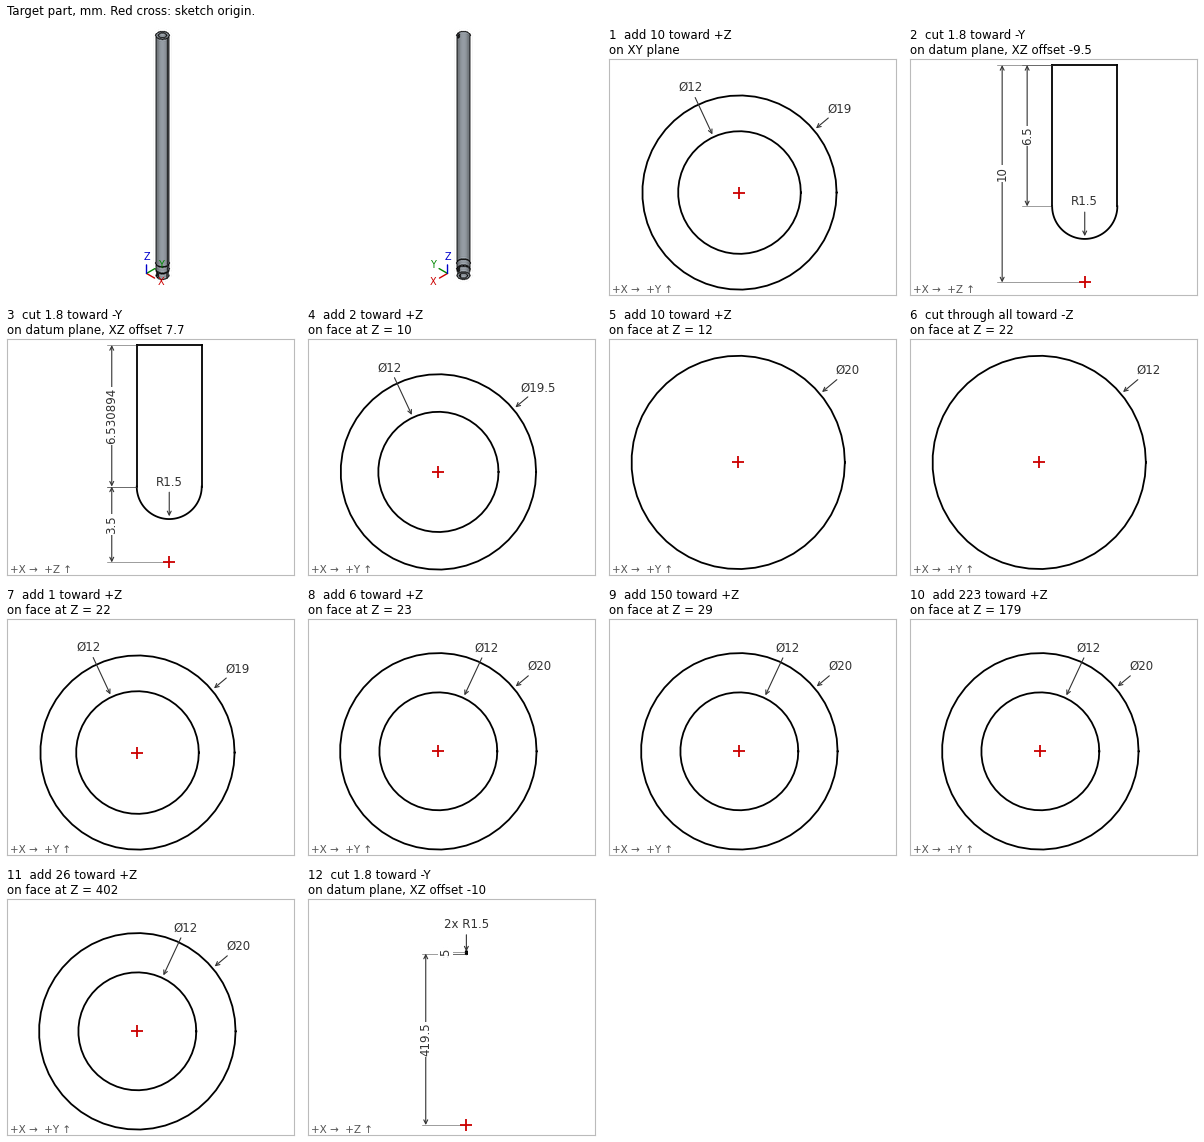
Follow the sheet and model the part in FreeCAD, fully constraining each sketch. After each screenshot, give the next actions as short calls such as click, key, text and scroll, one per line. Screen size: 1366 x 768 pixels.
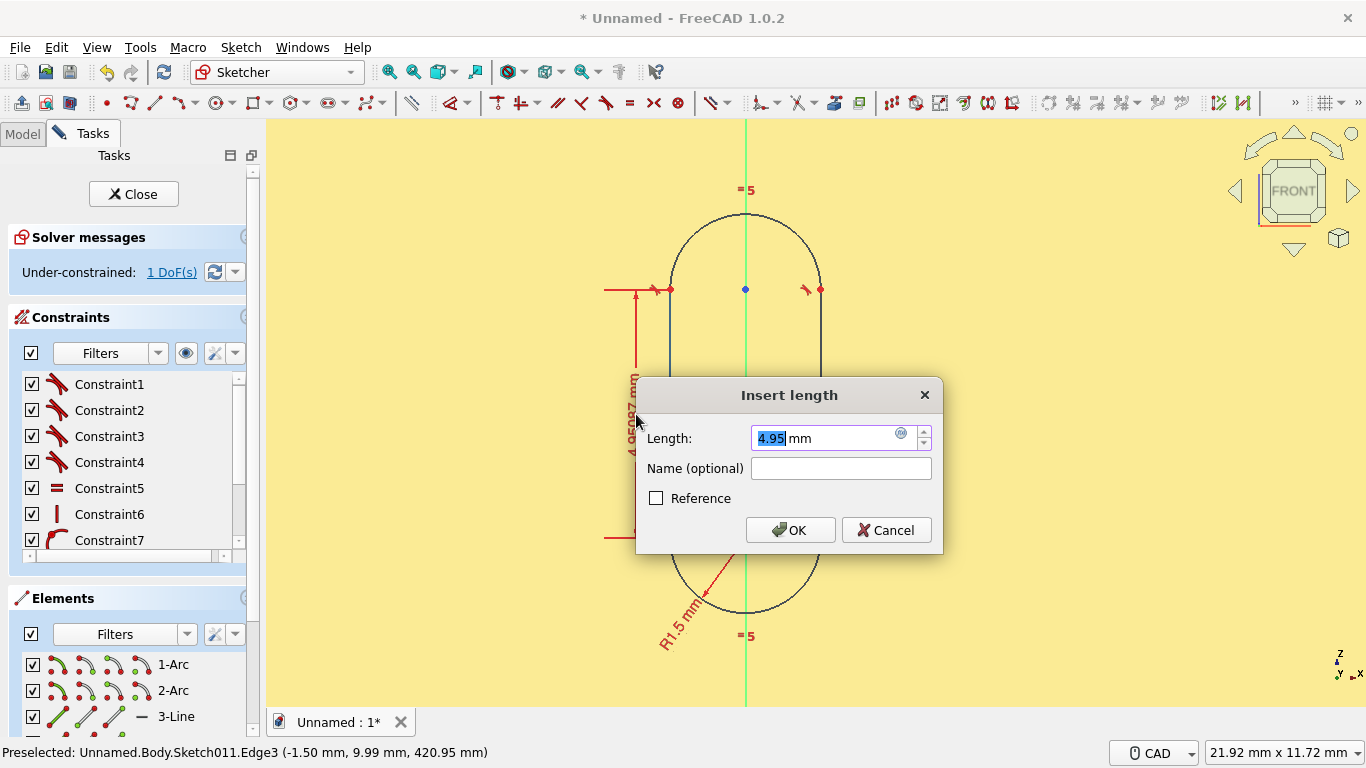
text(5)
key(Return)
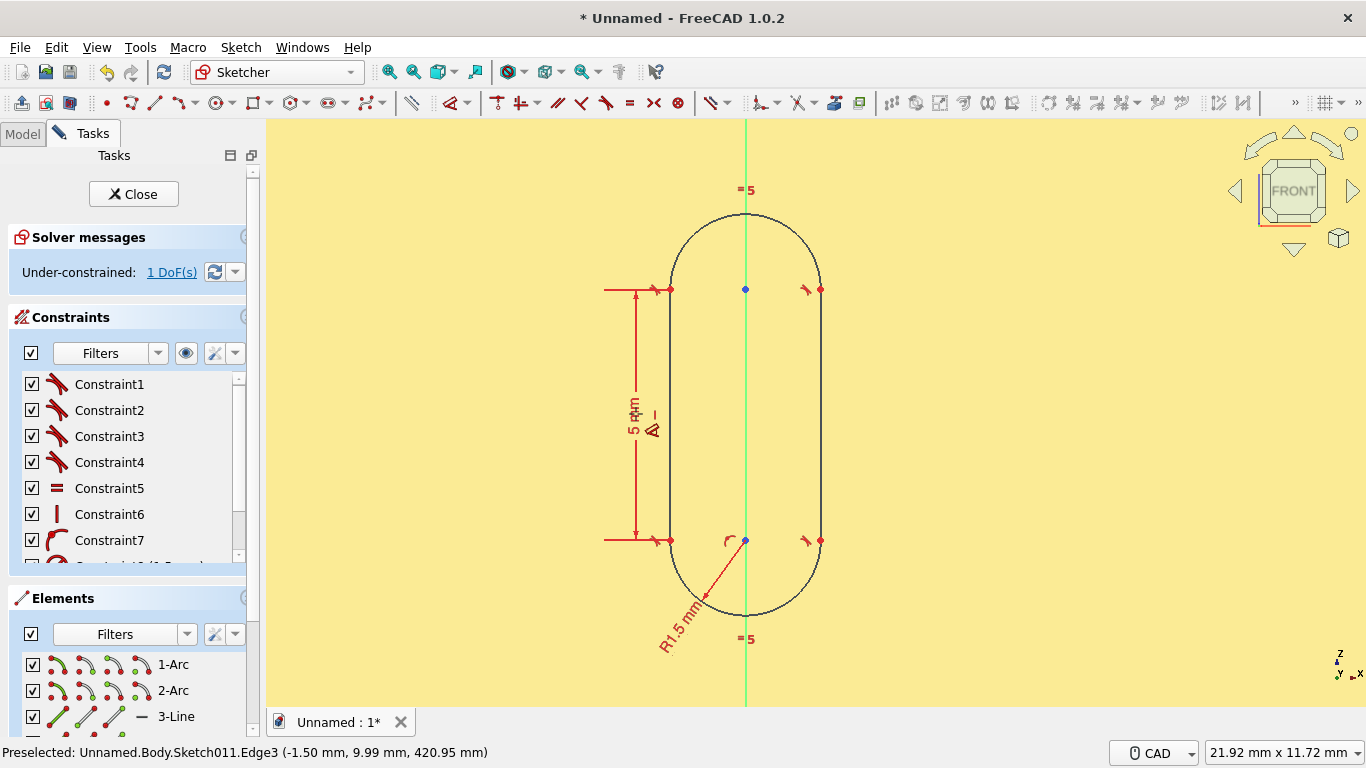
click(670, 540)
click(636, 578)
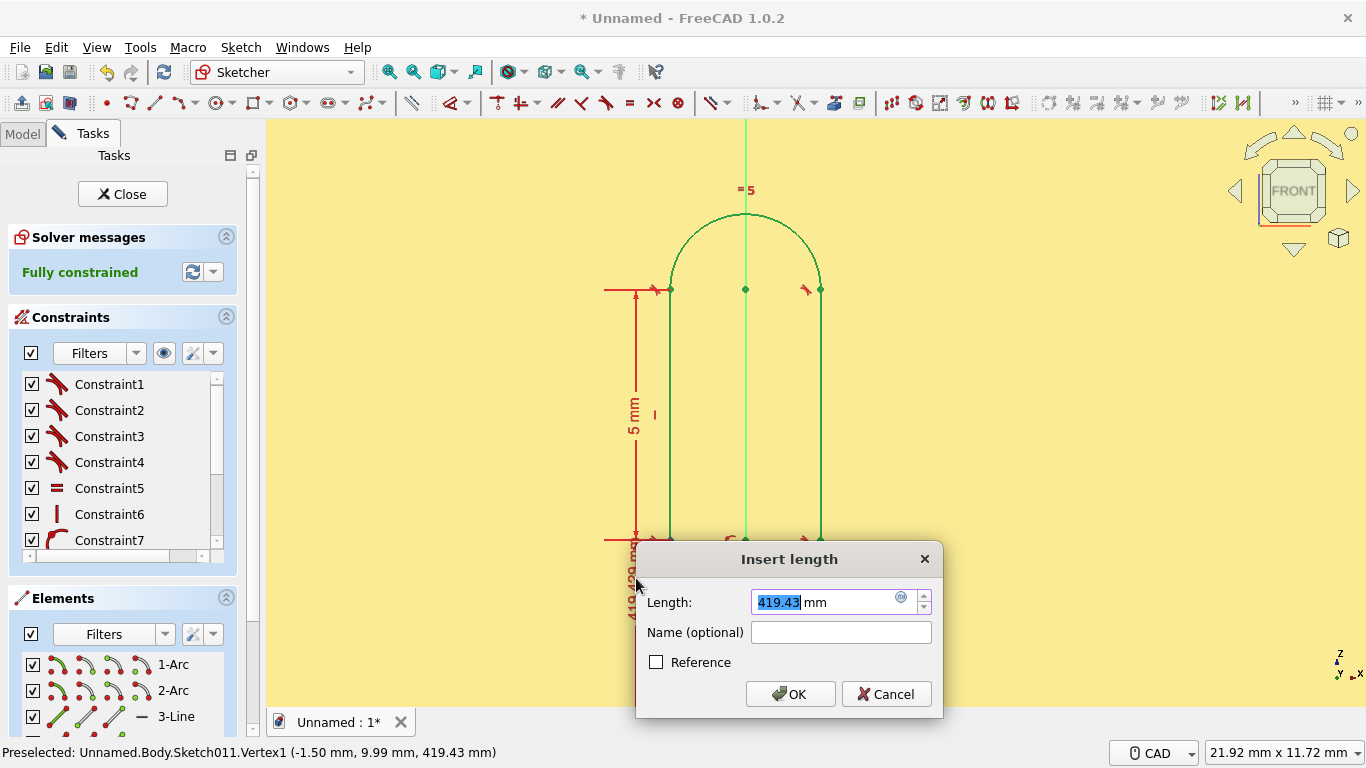
text(419.5)
key(Return)
key(Escape)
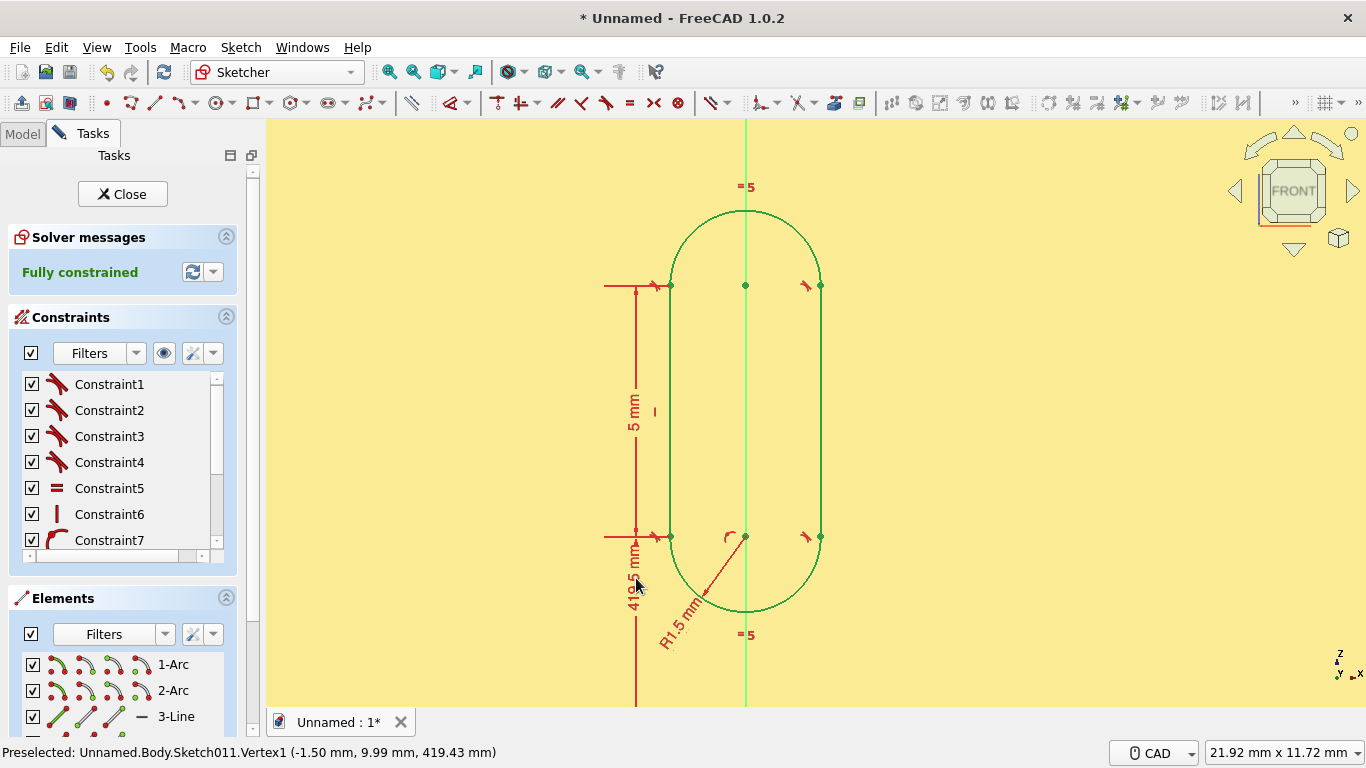
click(123, 194)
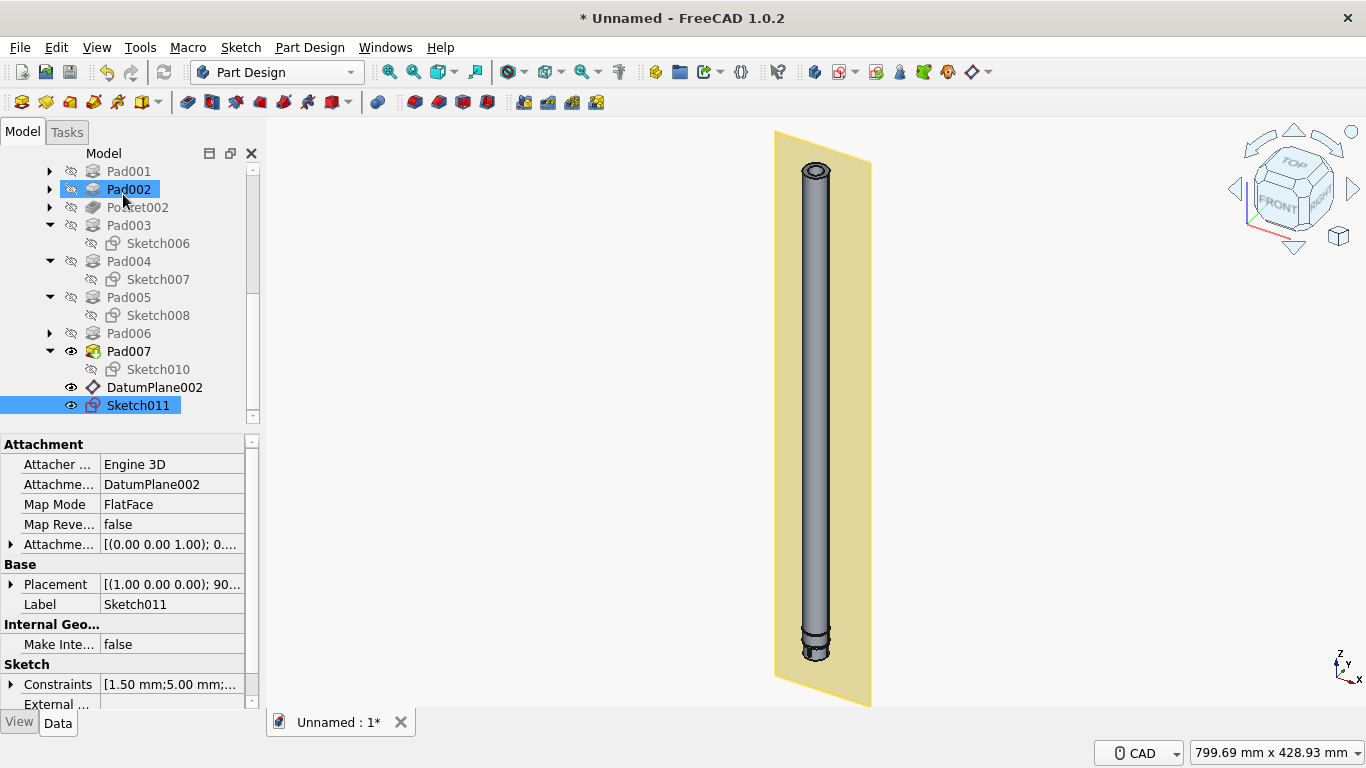
click(188, 102)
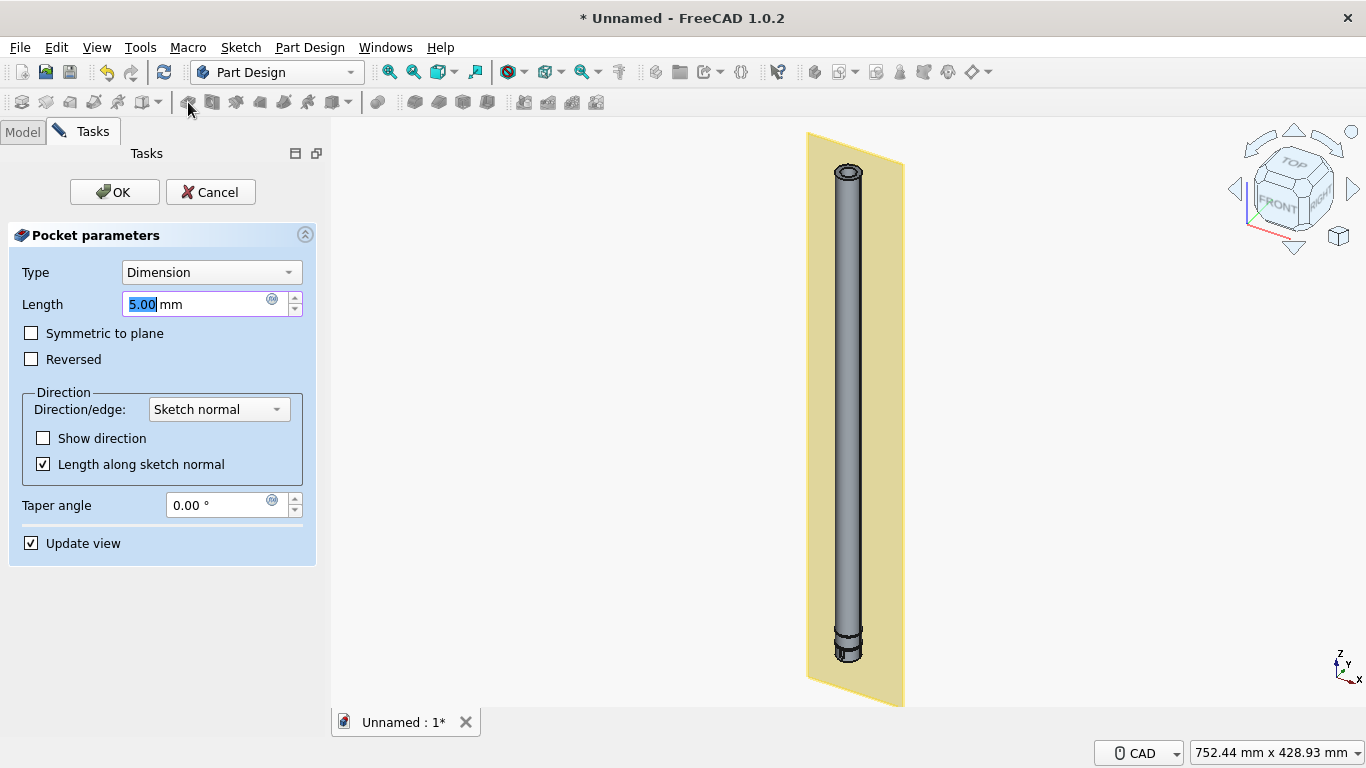
text(1.8)
key(Tab)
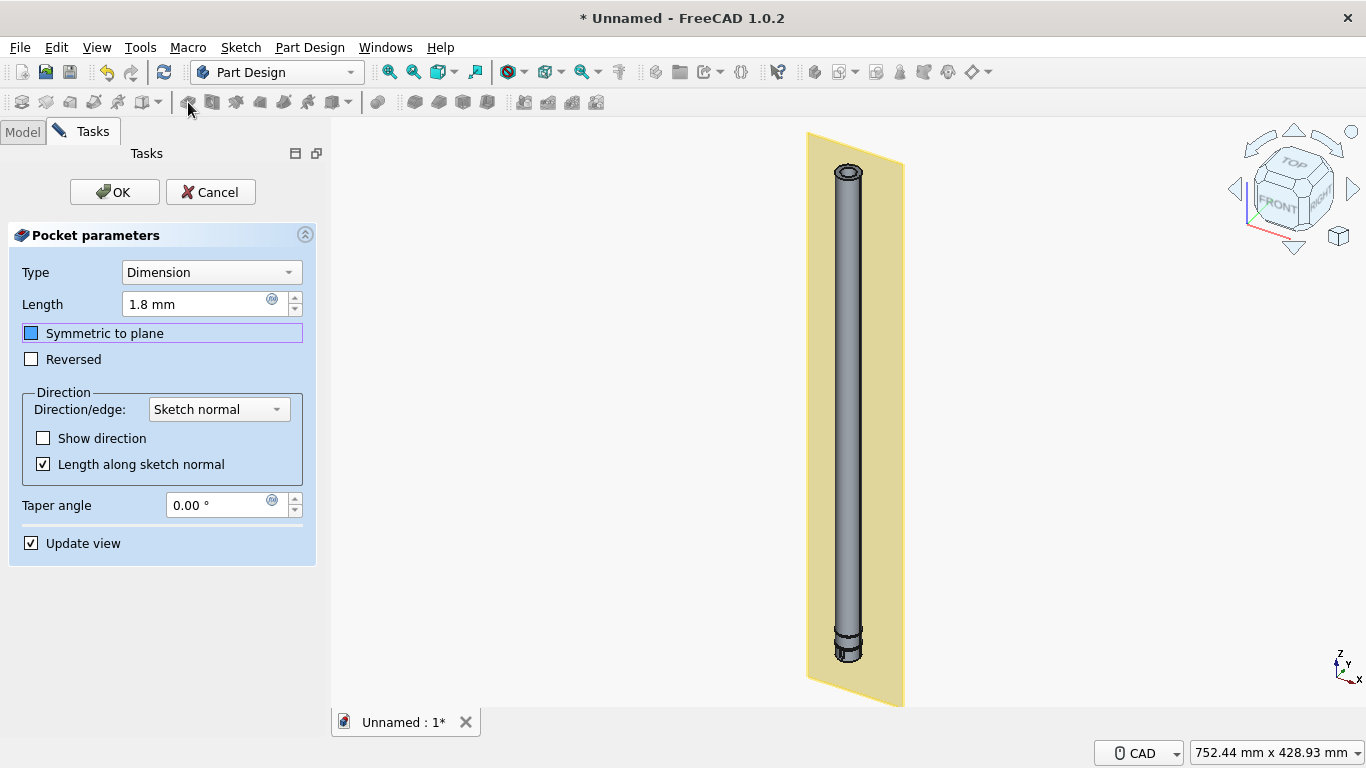
click(30, 359)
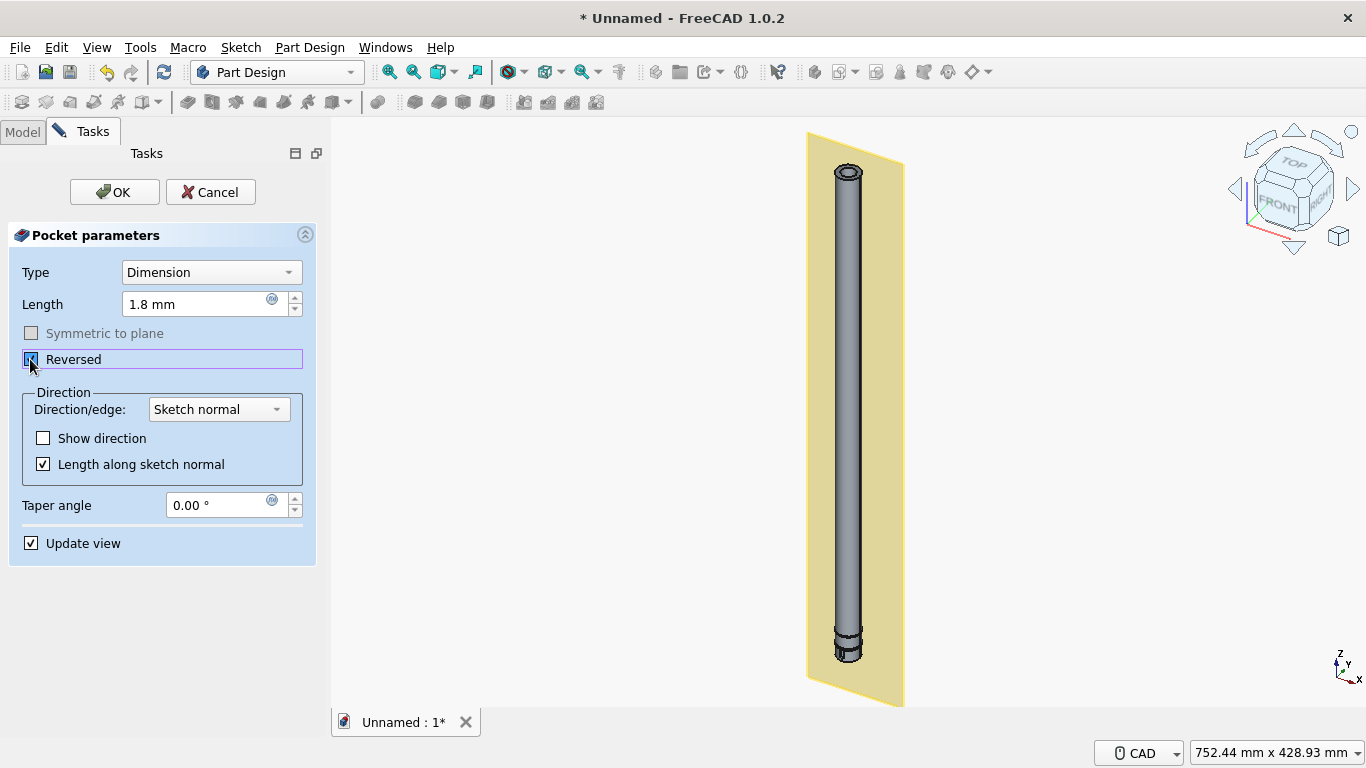
click(115, 192)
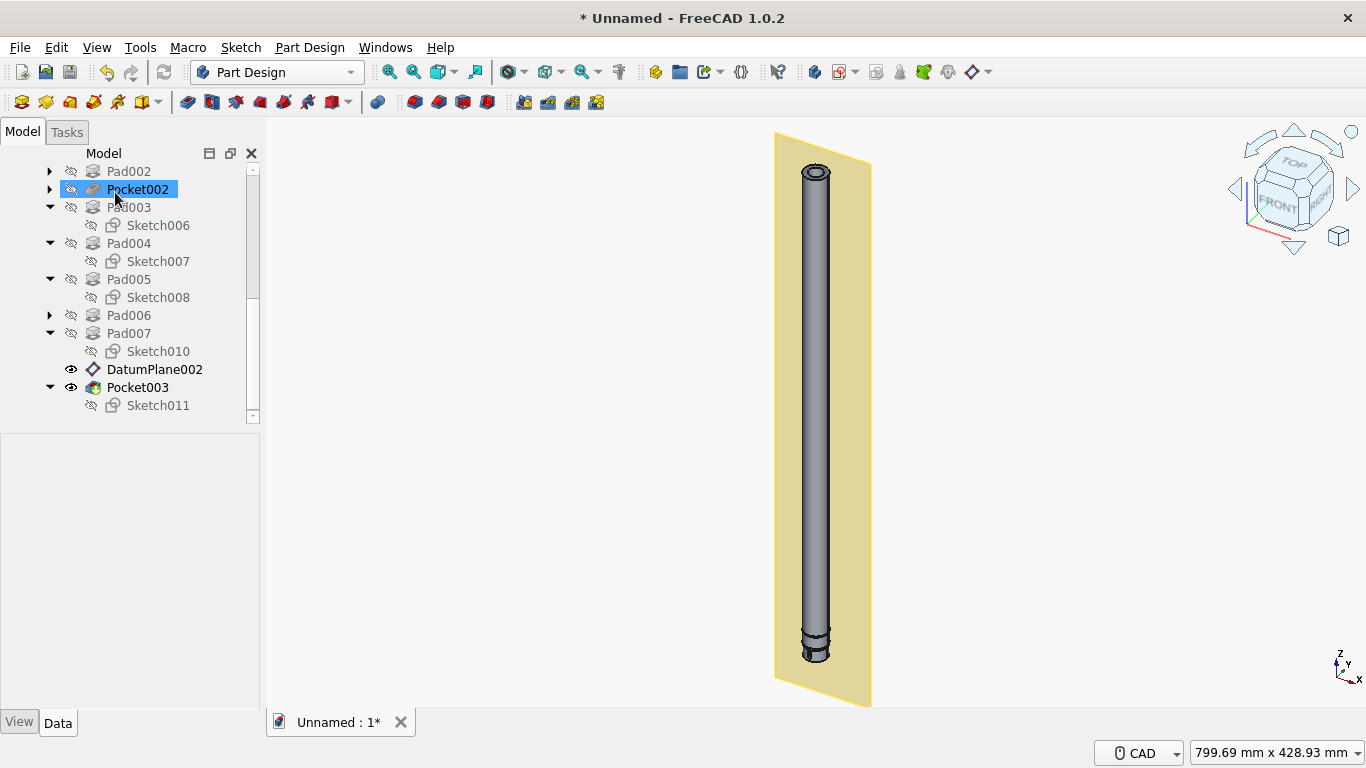
click(116, 369)
key(space)